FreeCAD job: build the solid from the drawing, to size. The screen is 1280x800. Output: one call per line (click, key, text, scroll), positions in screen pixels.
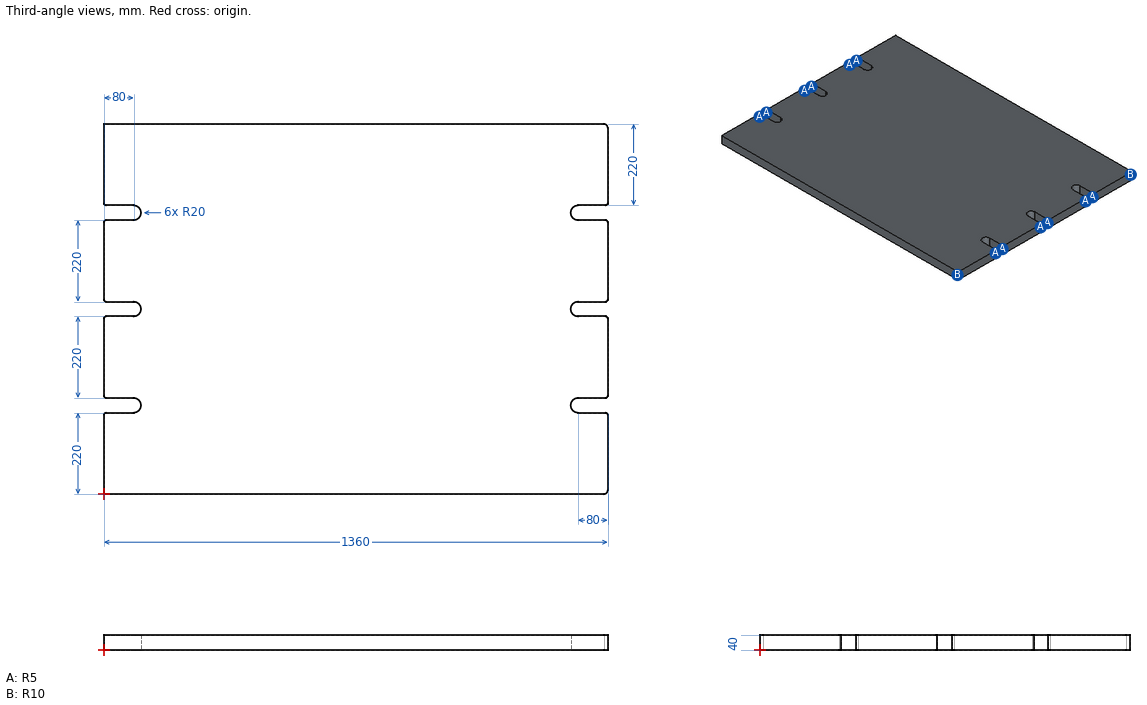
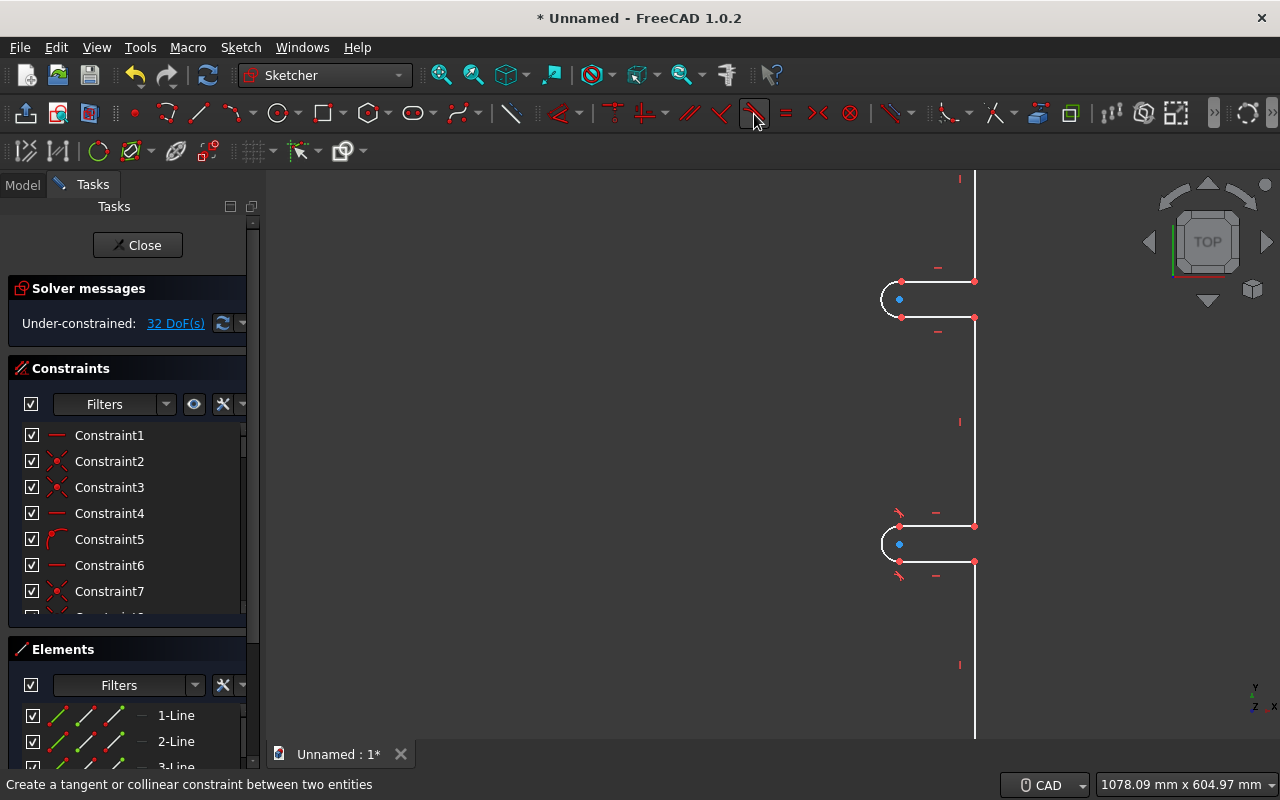
click(953, 317)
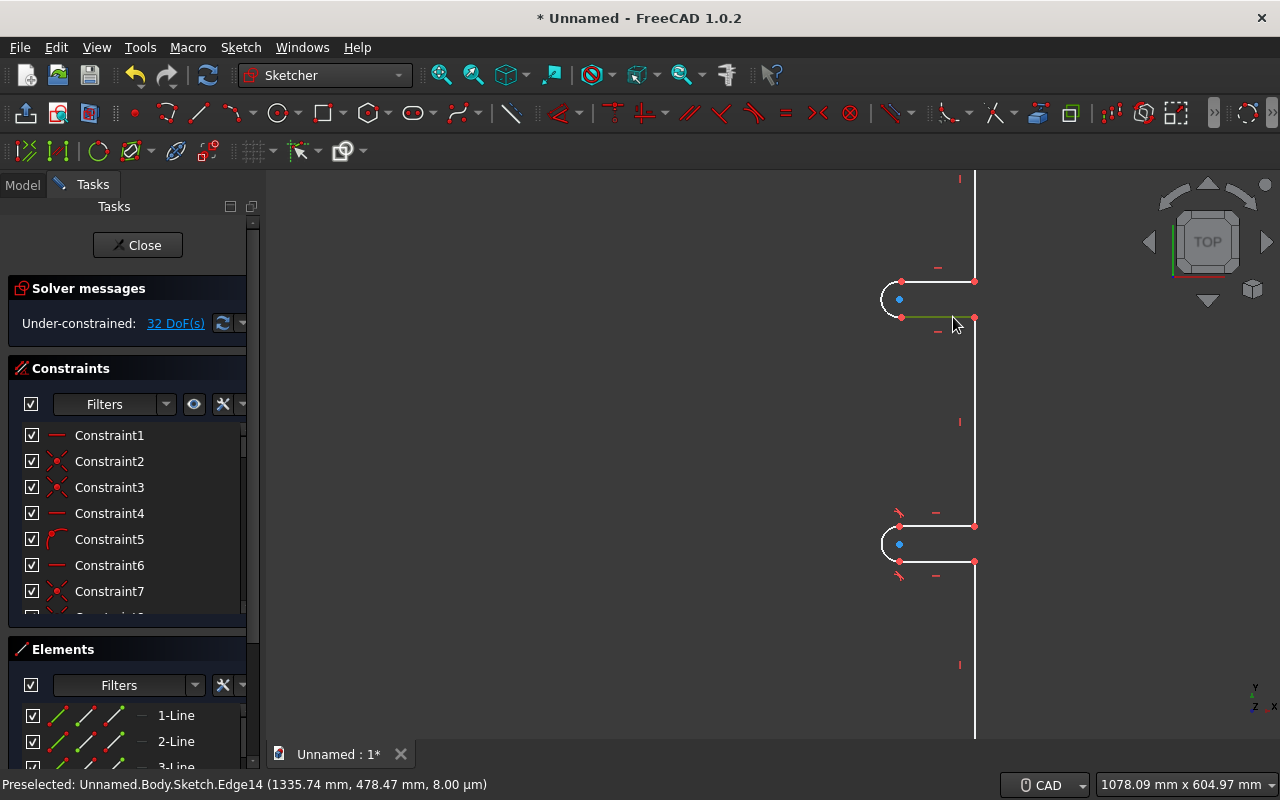
click(885, 288)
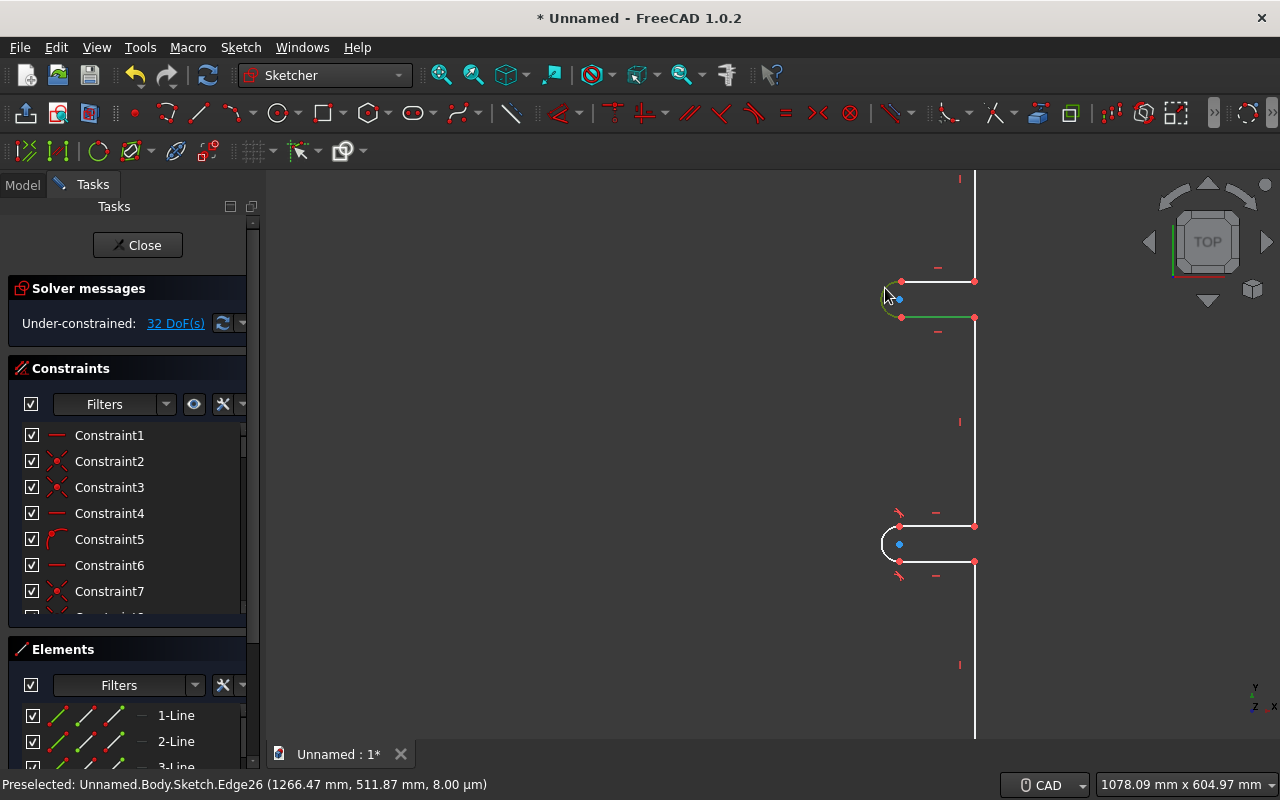
click(754, 114)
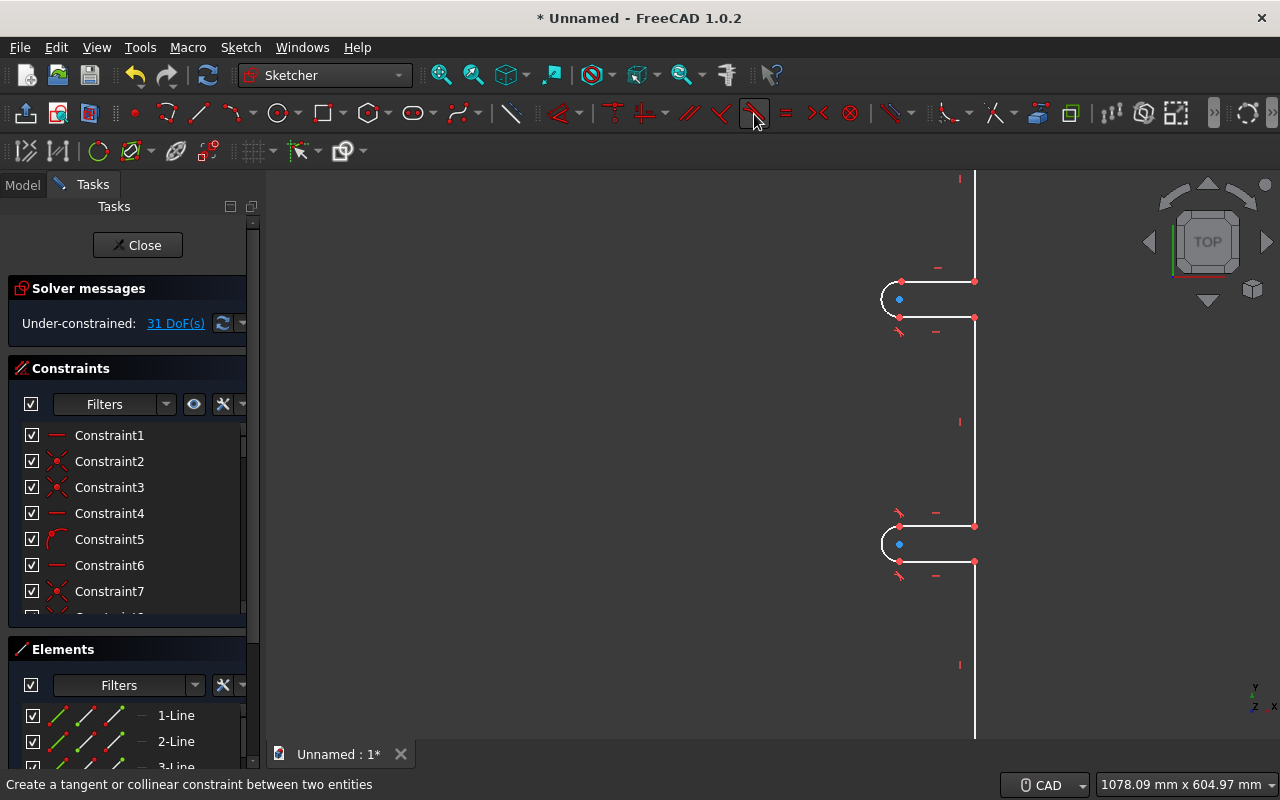
click(923, 282)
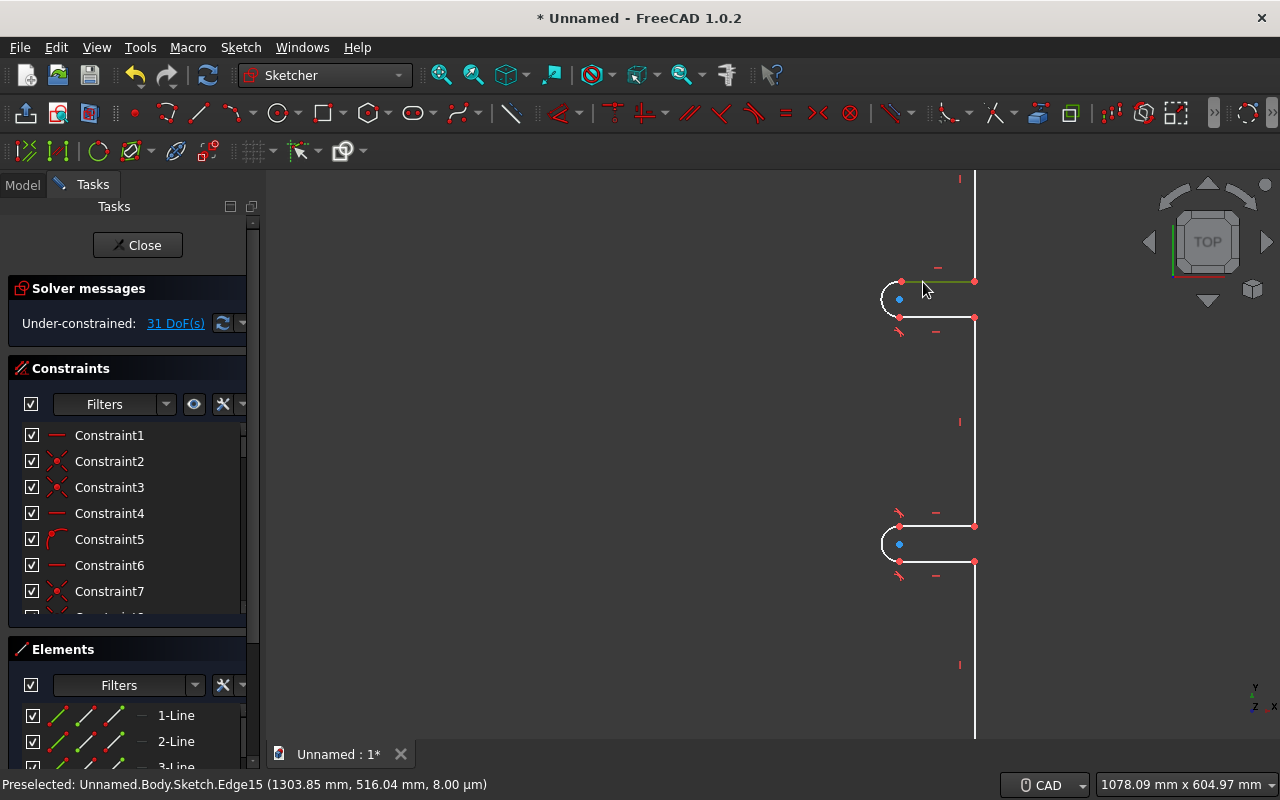
click(886, 288)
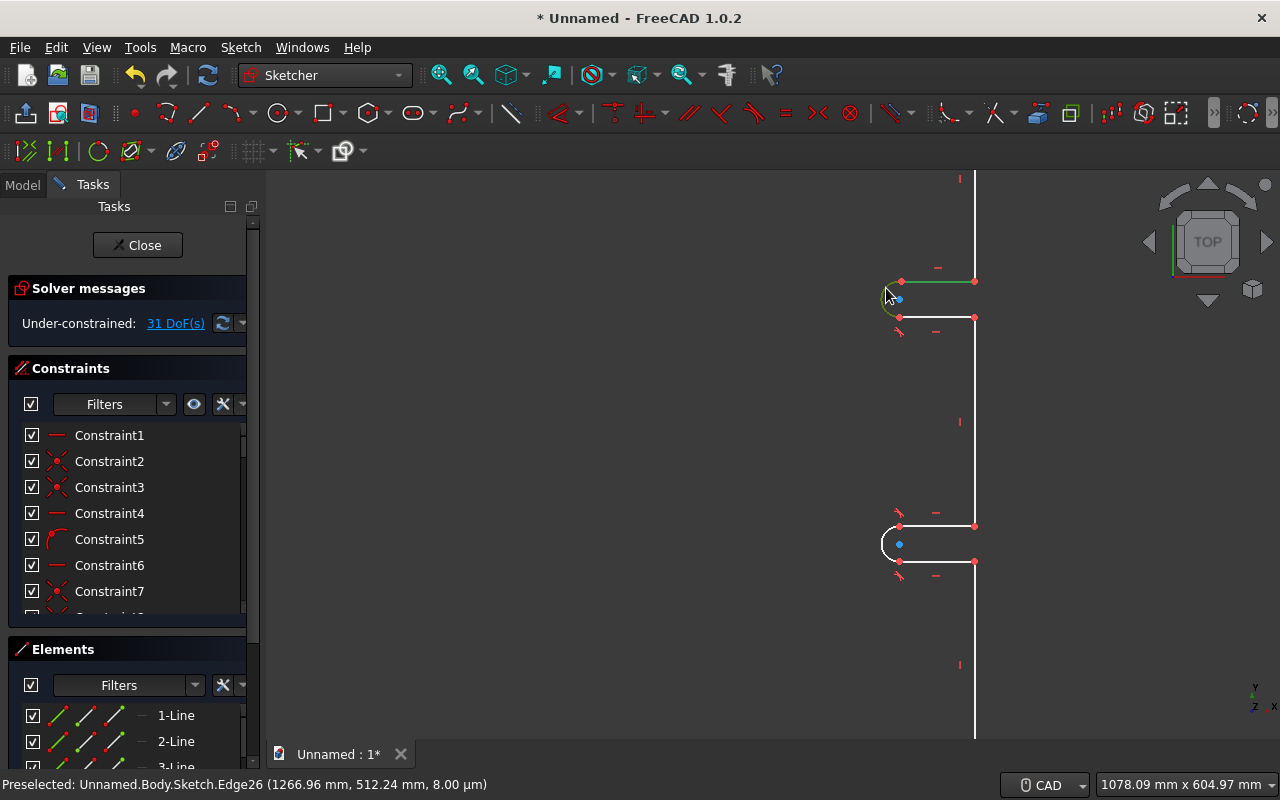
click(754, 114)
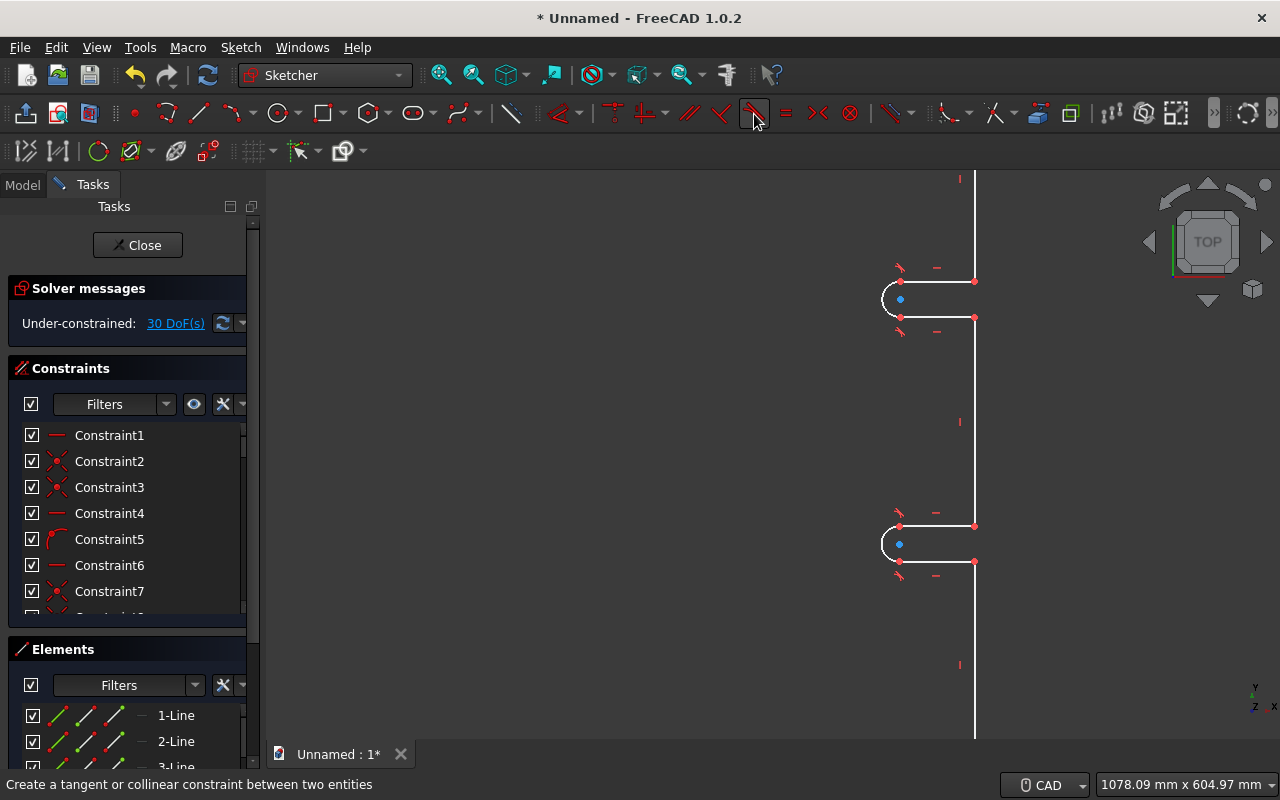
scroll(919, 546, down, 5)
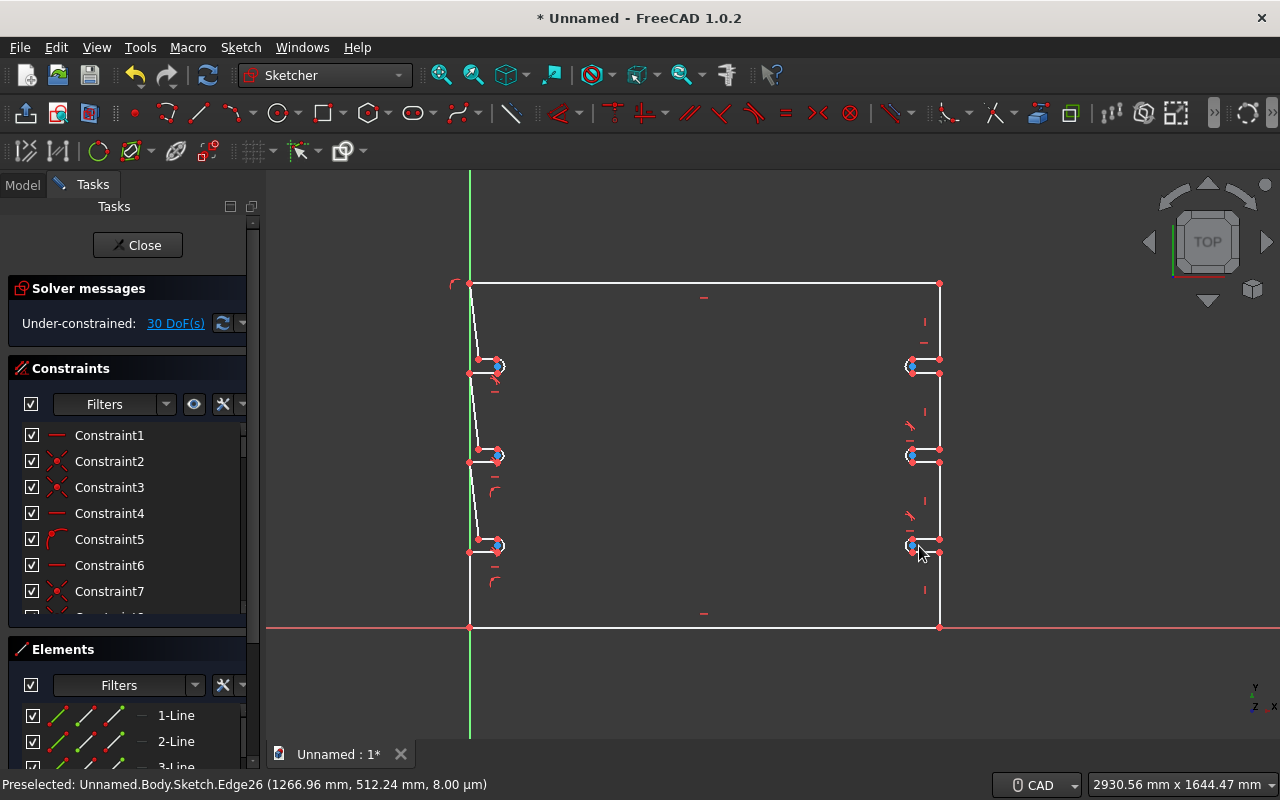
scroll(932, 373, up, 3)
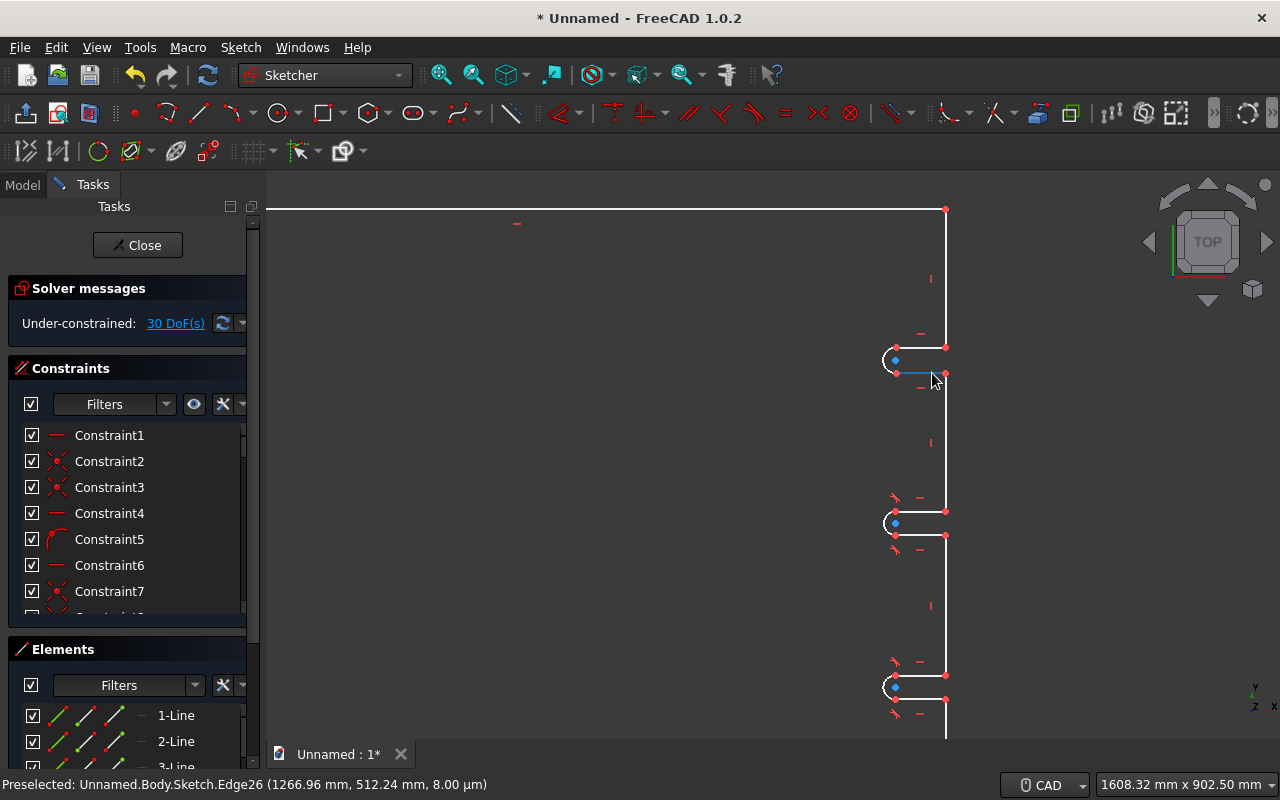
click(931, 373)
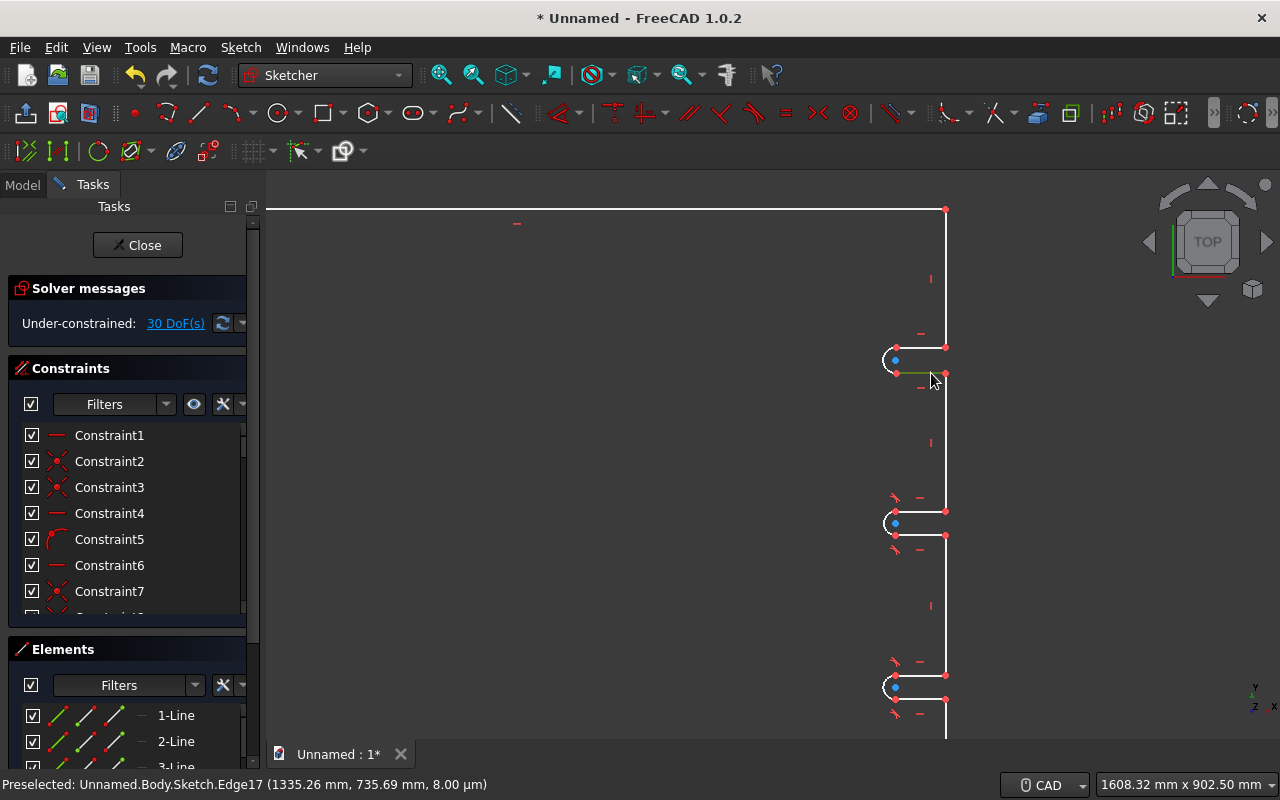
click(886, 353)